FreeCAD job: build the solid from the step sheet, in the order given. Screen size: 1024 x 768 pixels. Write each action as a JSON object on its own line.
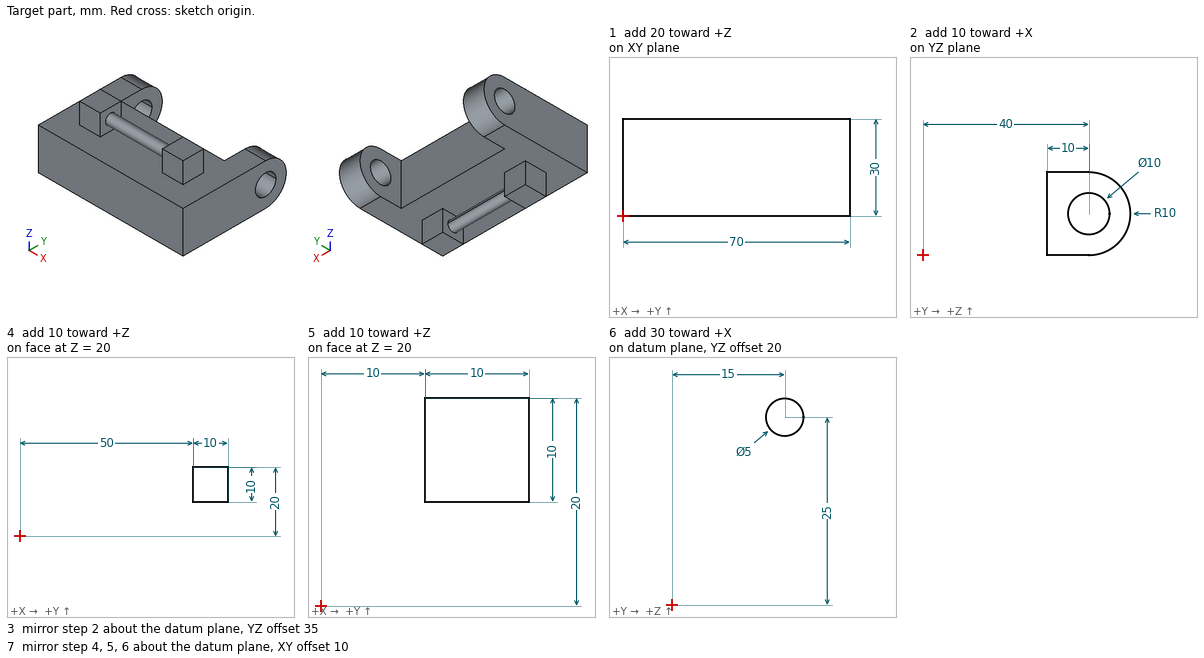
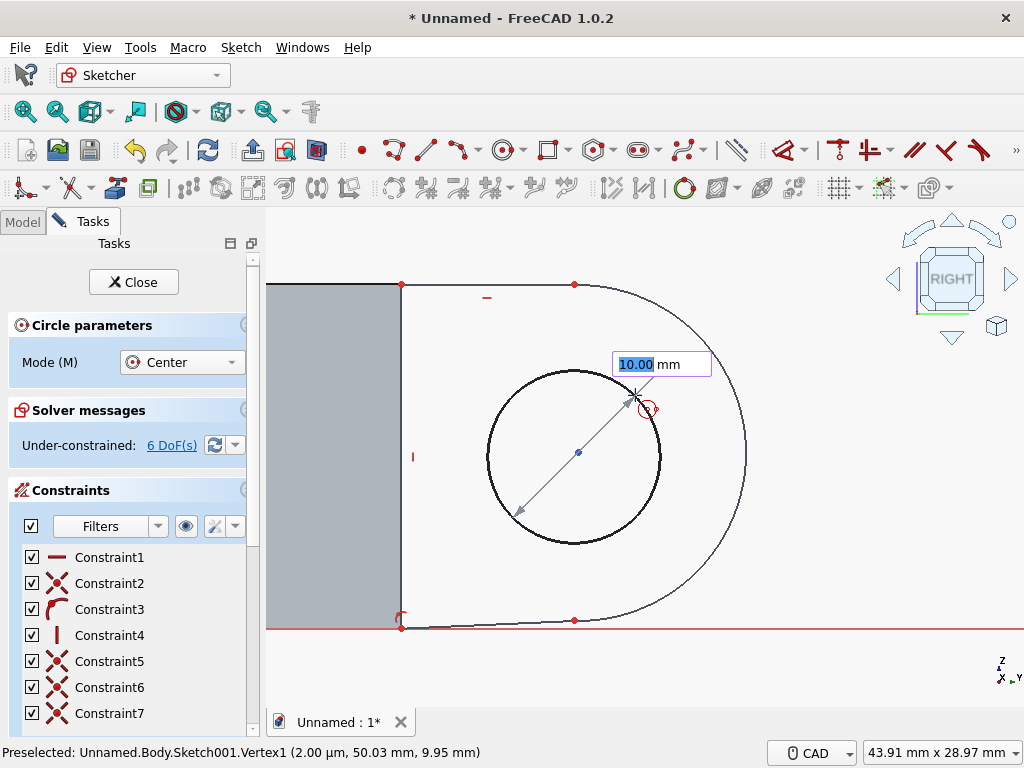
{"action": "type", "text": "10"}
{"action": "key", "text": "Return"}
{"action": "key", "text": "Escape"}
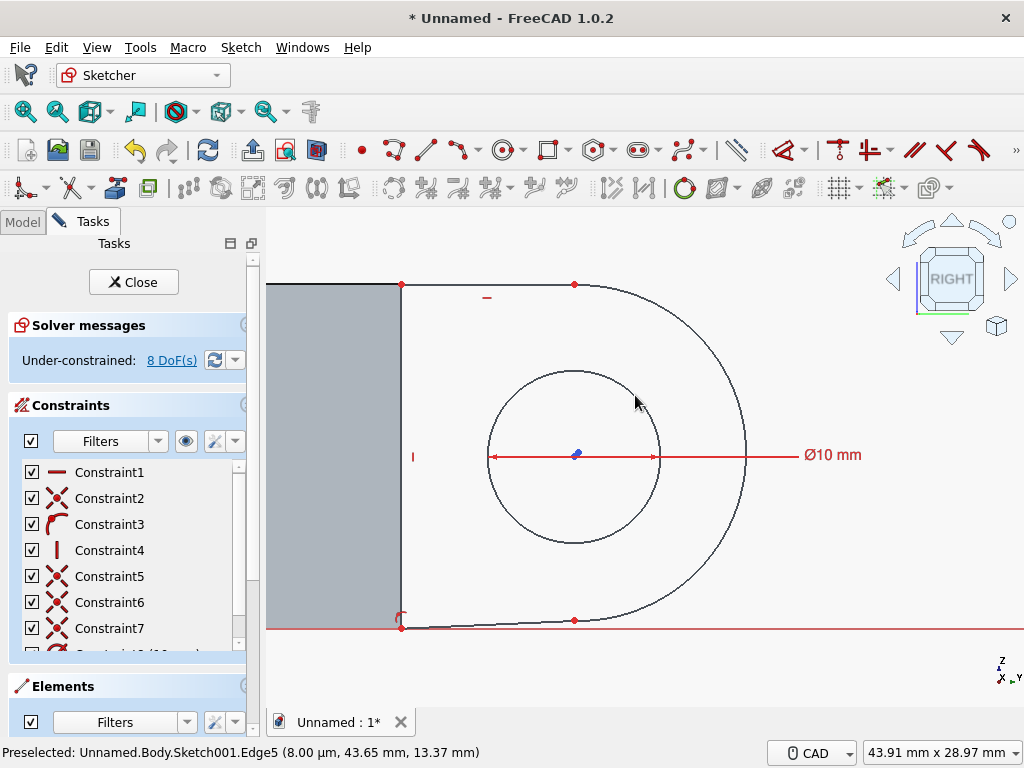
{"action": "left_click", "coordinate": [522, 285]}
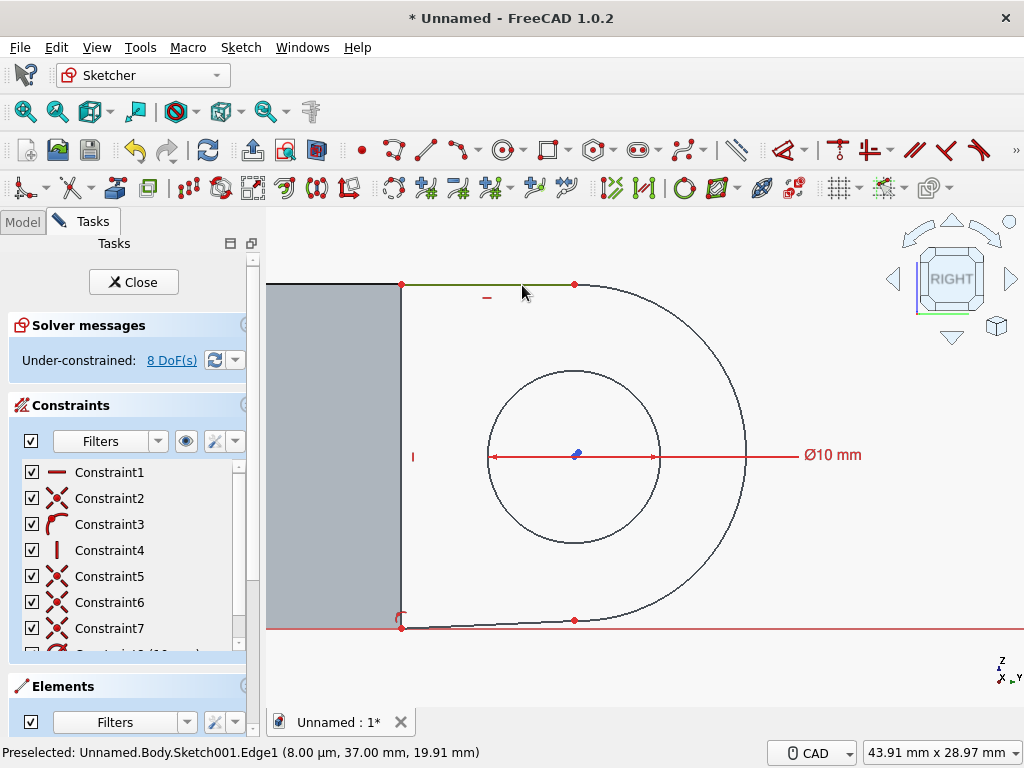
{"action": "left_click", "coordinate": [713, 553]}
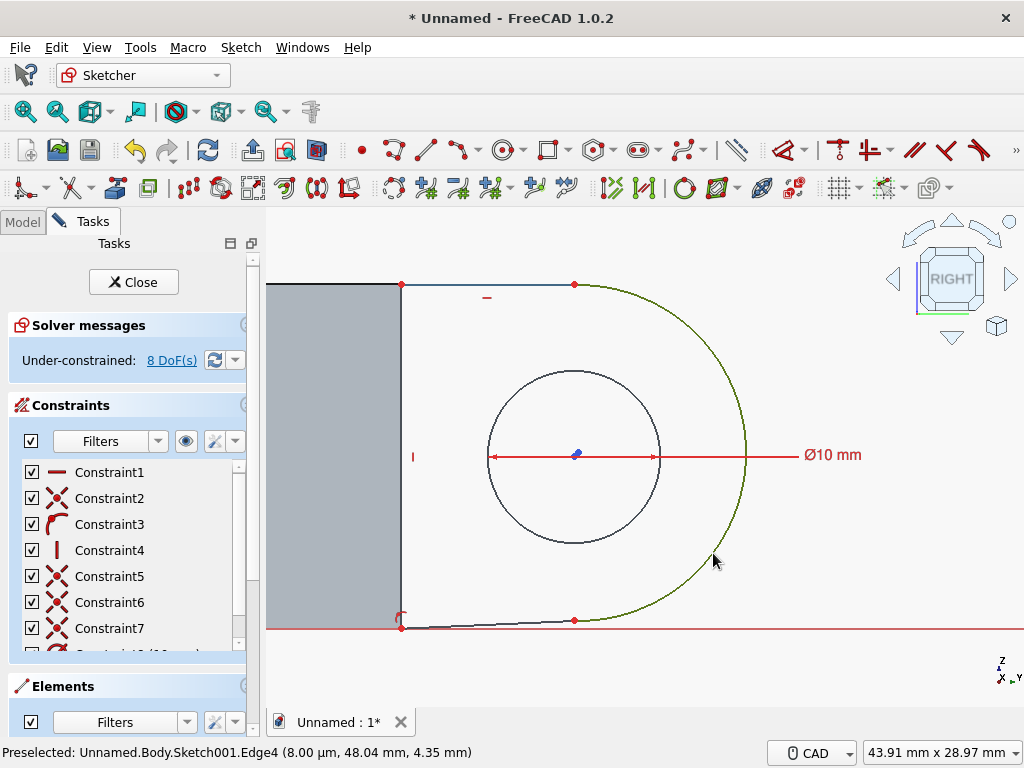
{"action": "key", "text": "t"}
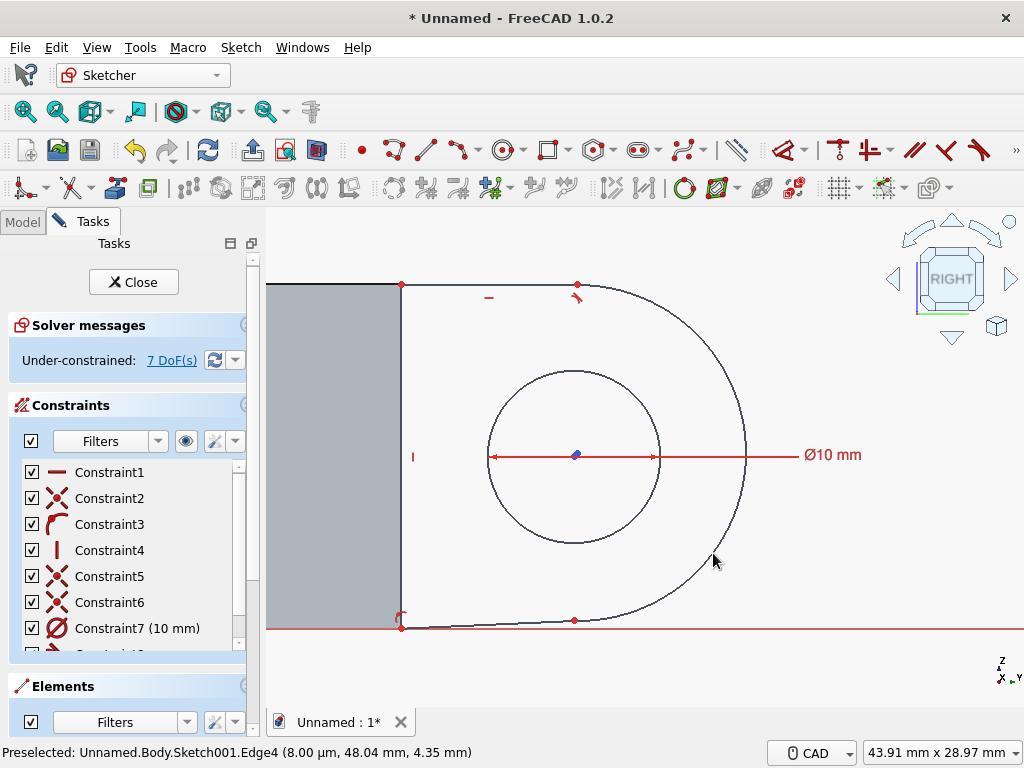
{"action": "left_click", "coordinate": [453, 626]}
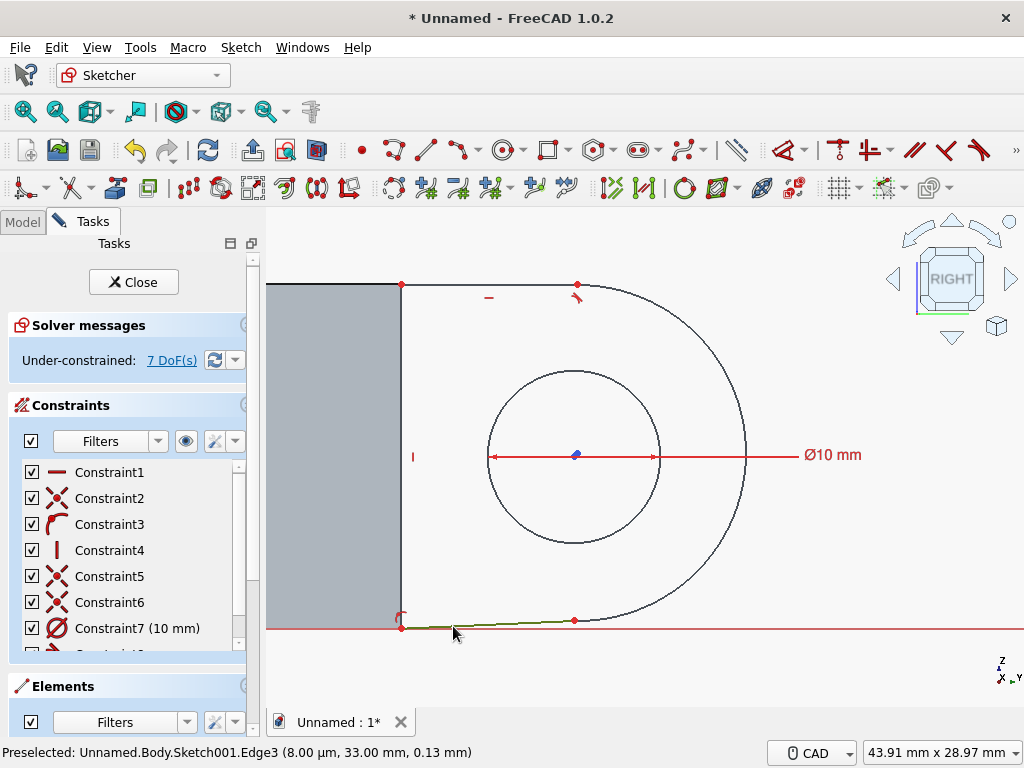
{"action": "left_click", "coordinate": [712, 554]}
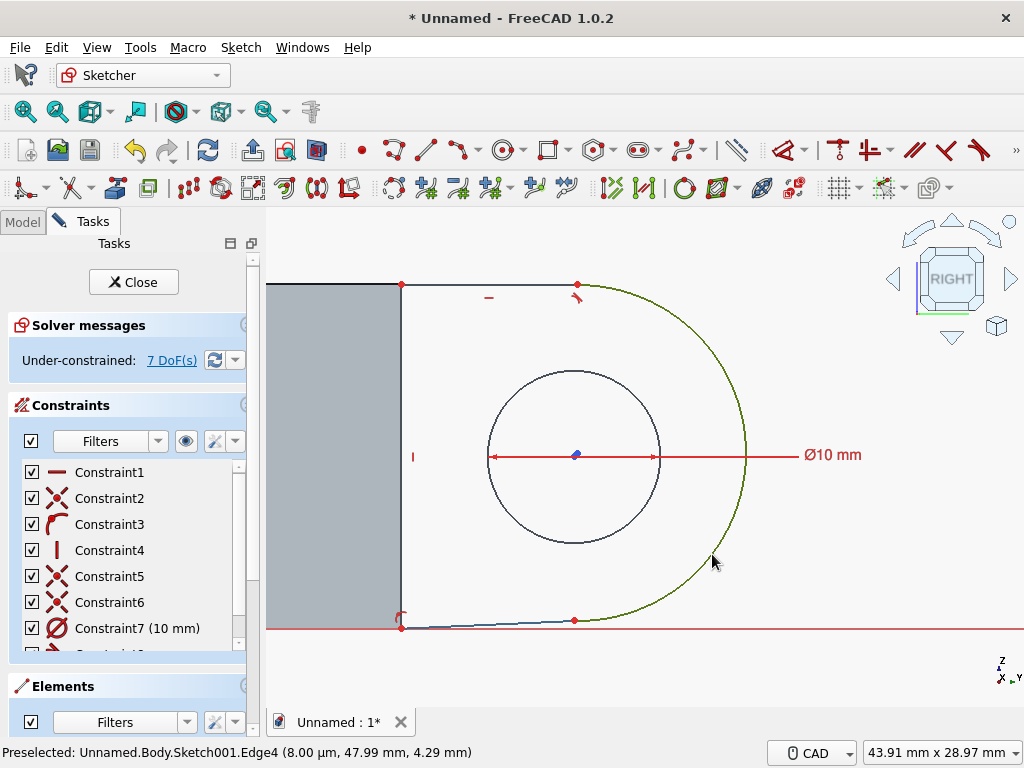
{"action": "key", "text": "t"}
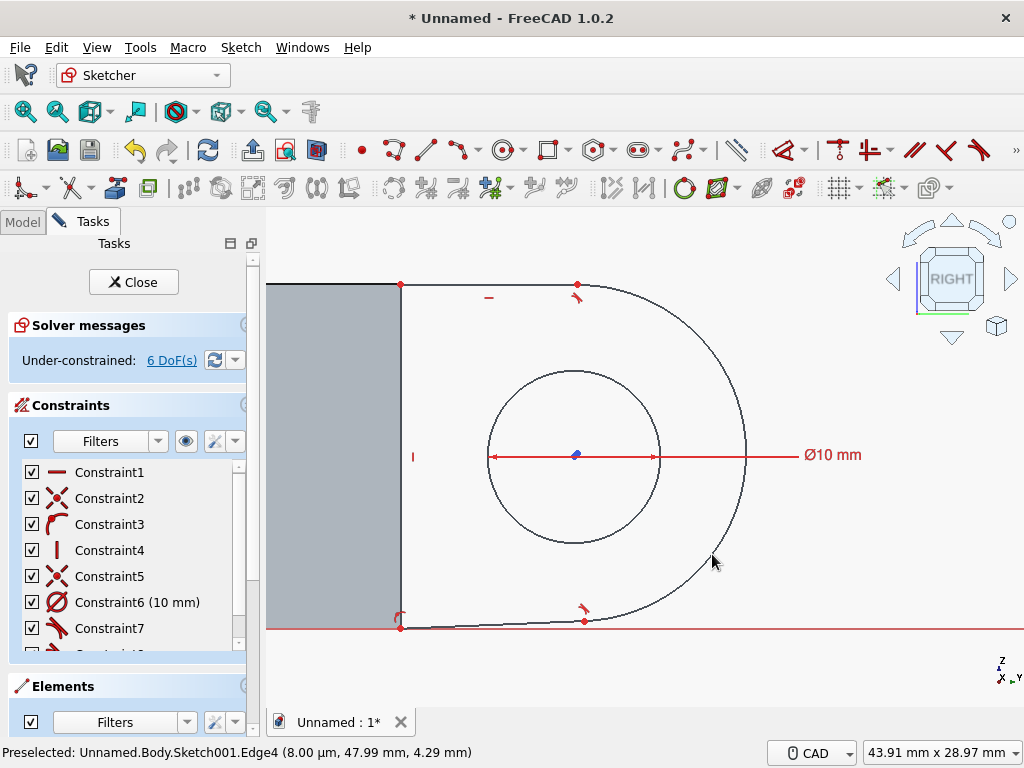
{"action": "left_click", "coordinate": [456, 626]}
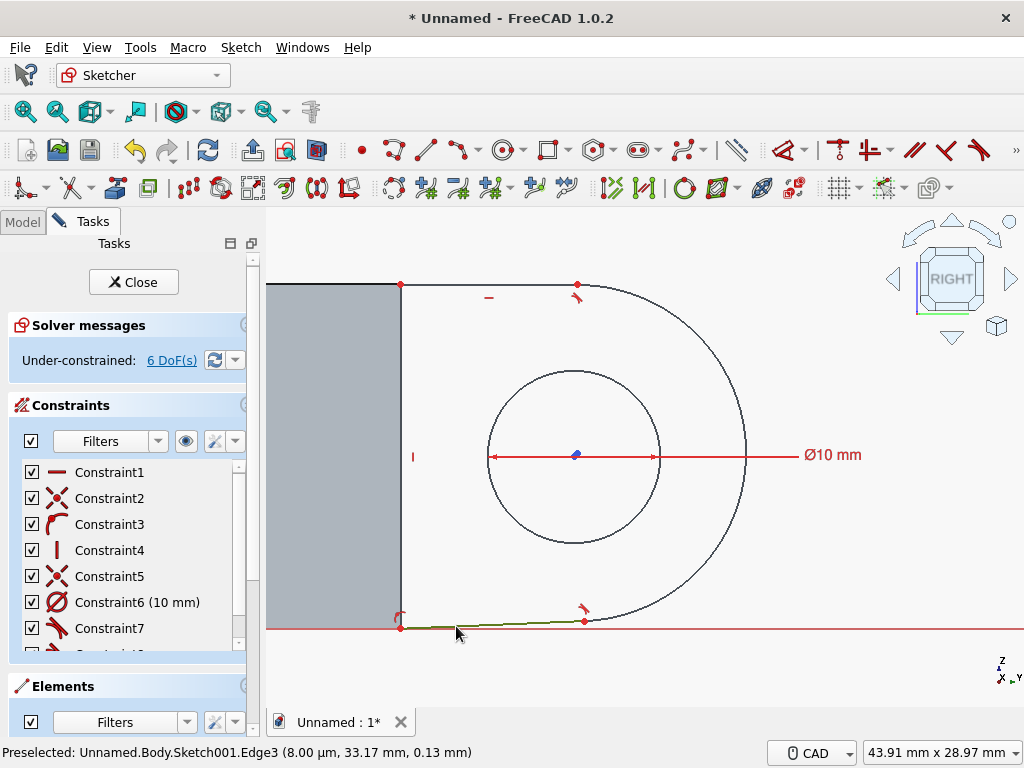
{"action": "key", "text": "h"}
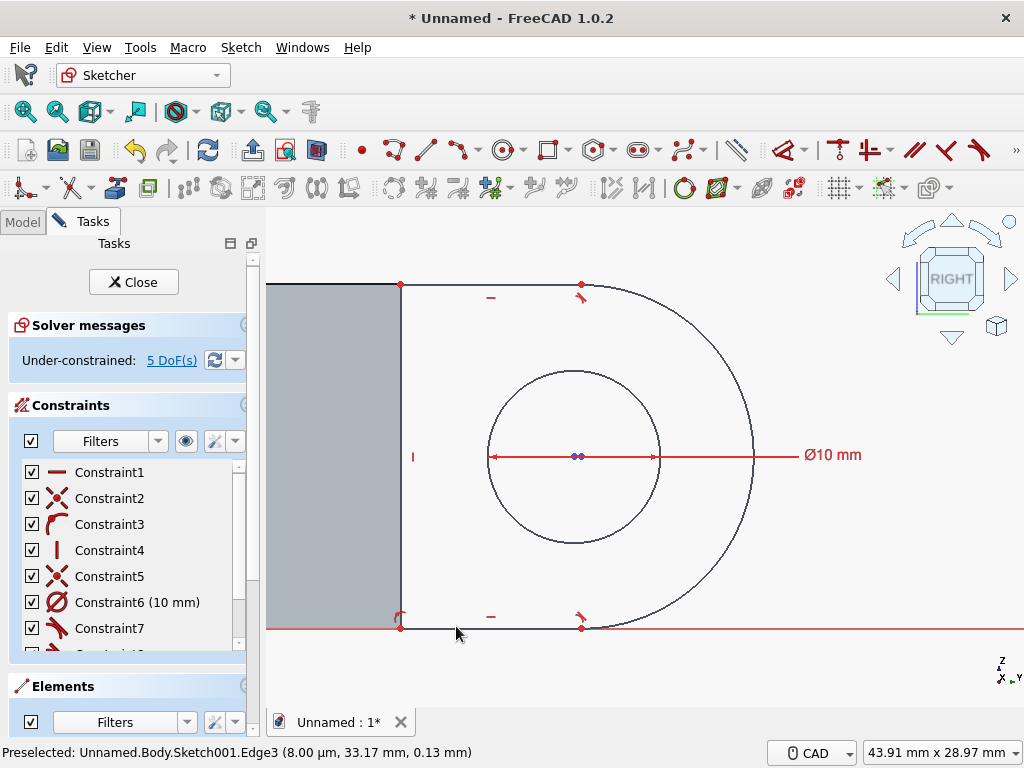
{"action": "left_click", "coordinate": [635, 396]}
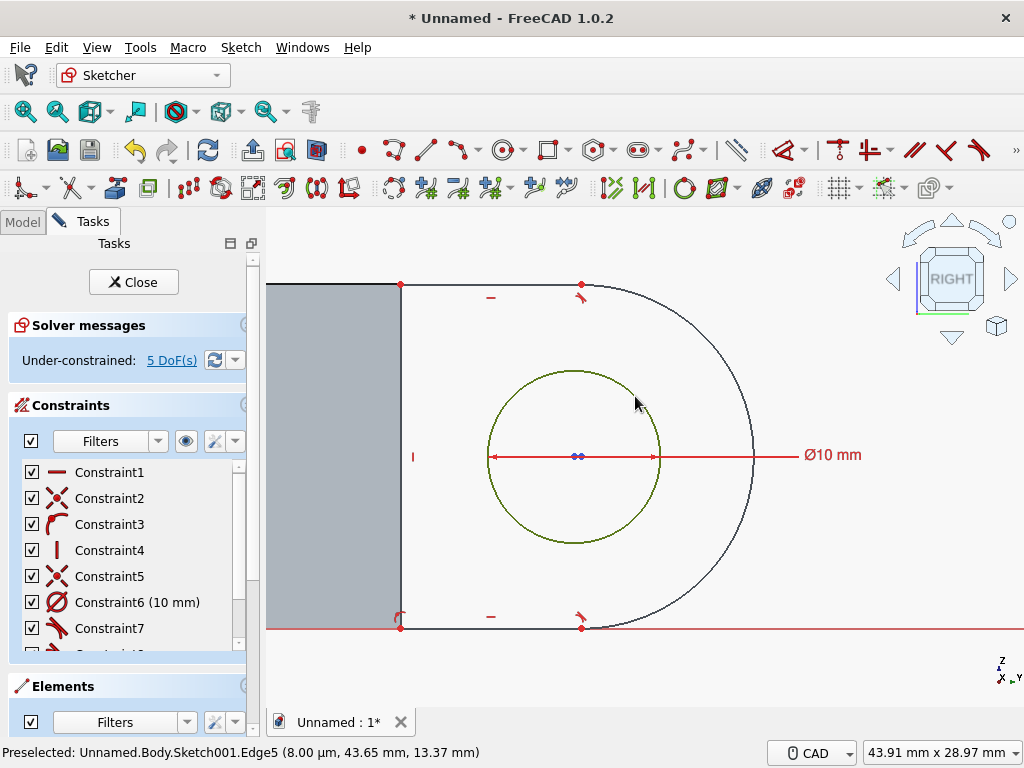
{"action": "left_click", "coordinate": [721, 558]}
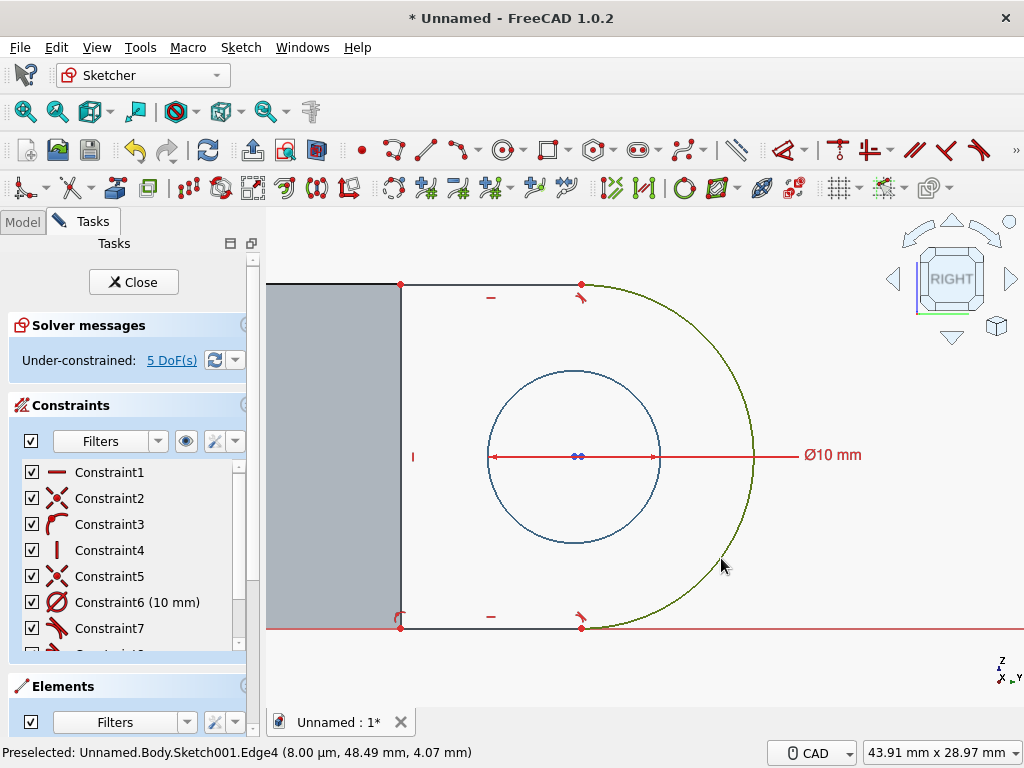
{"action": "key", "text": "c"}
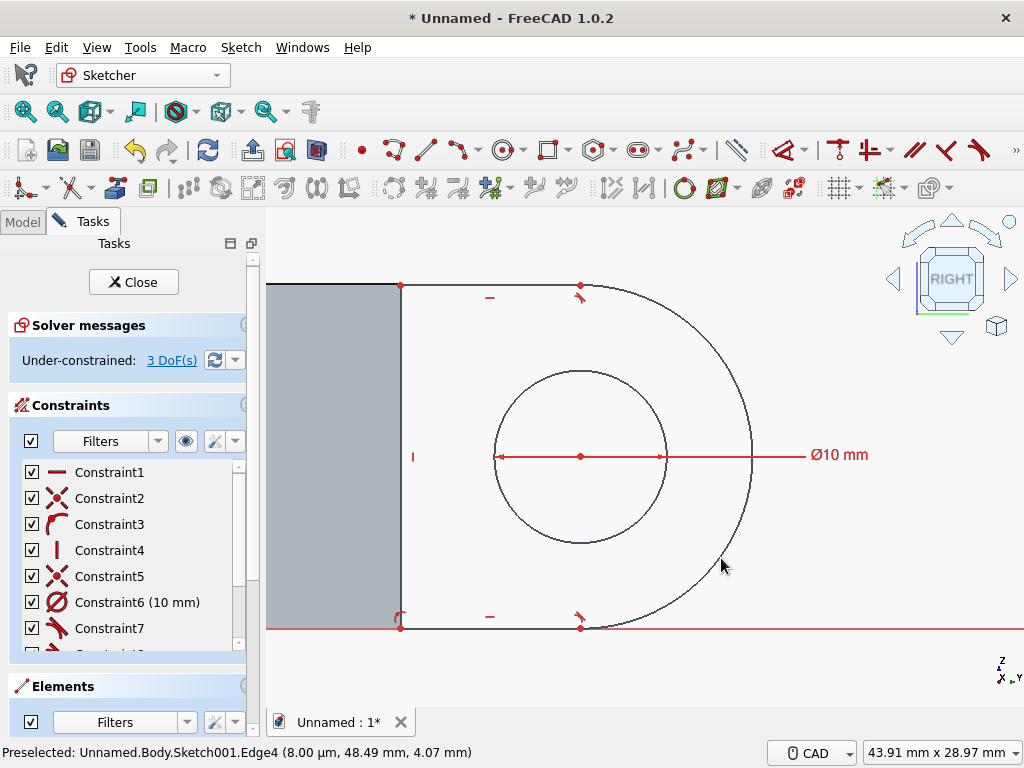
{"action": "left_click", "coordinate": [784, 150]}